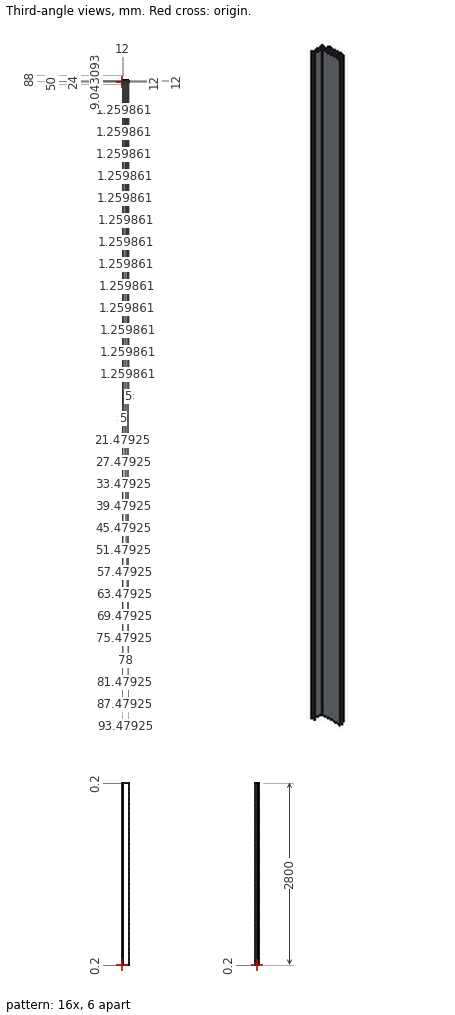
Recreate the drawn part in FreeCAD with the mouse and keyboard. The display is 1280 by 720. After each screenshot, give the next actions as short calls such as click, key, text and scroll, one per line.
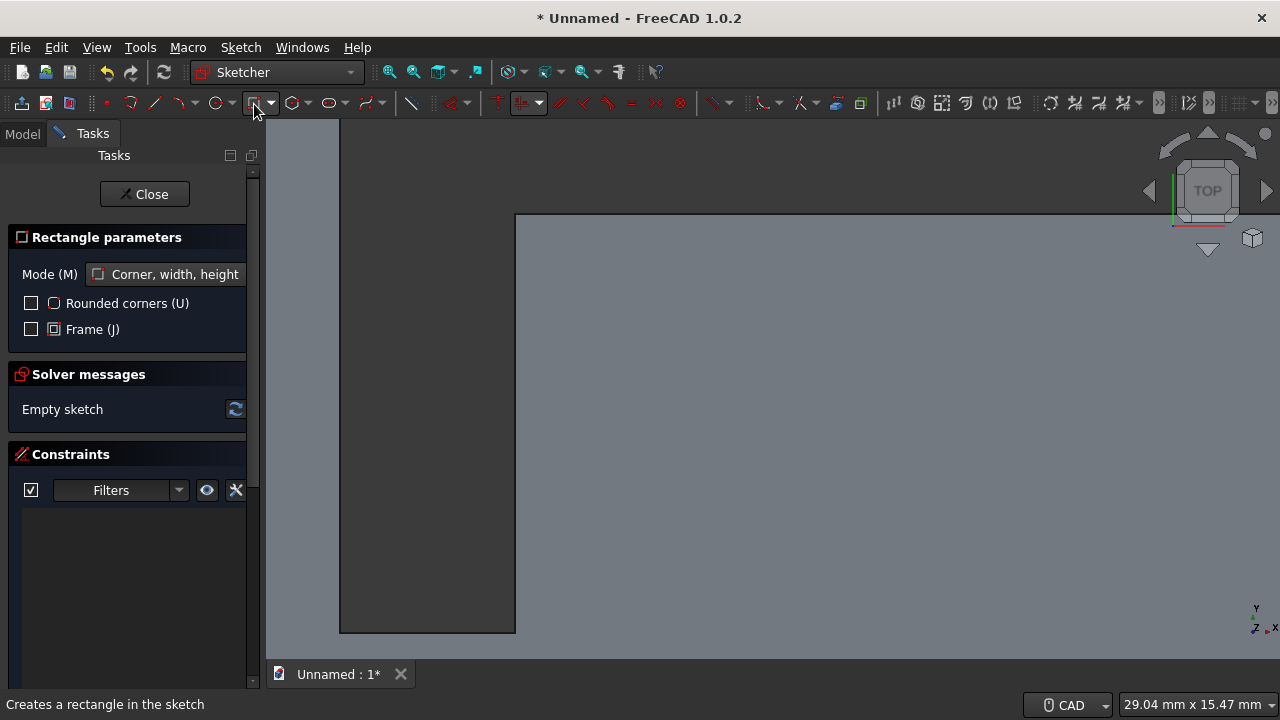
click(671, 214)
move(715, 530)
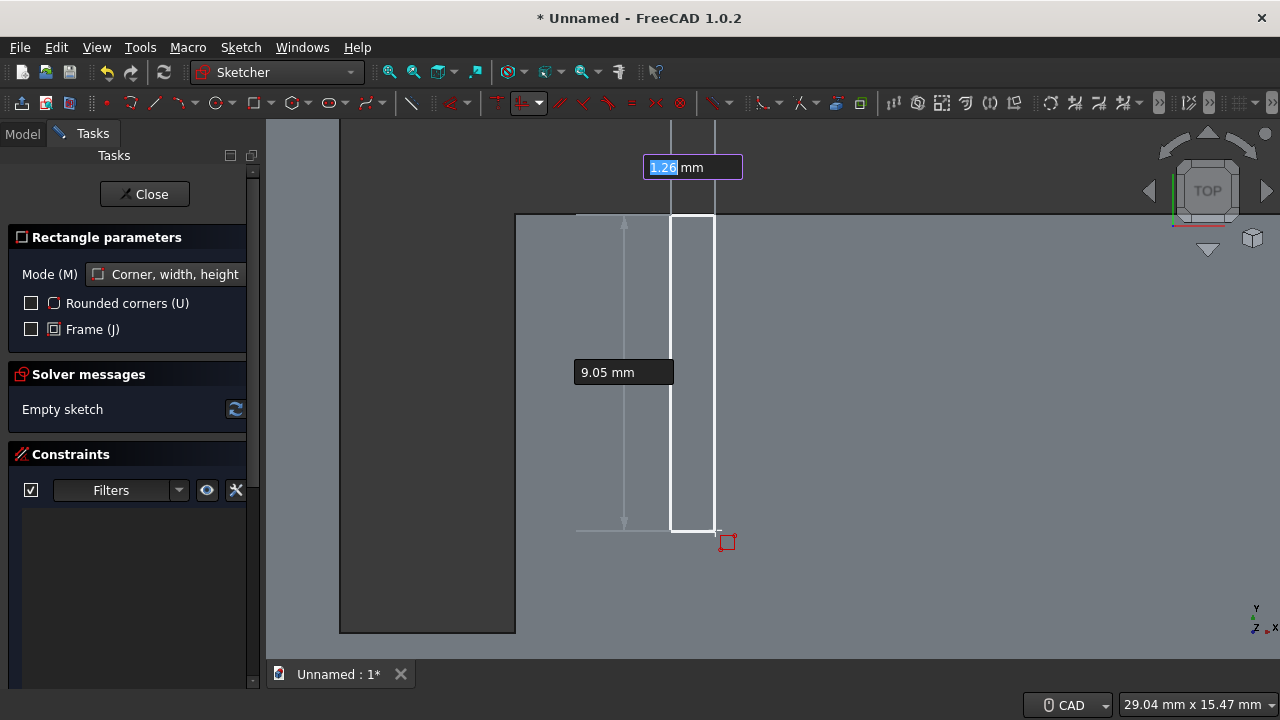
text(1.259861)
key(Tab)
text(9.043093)
key(Return)
key(Escape)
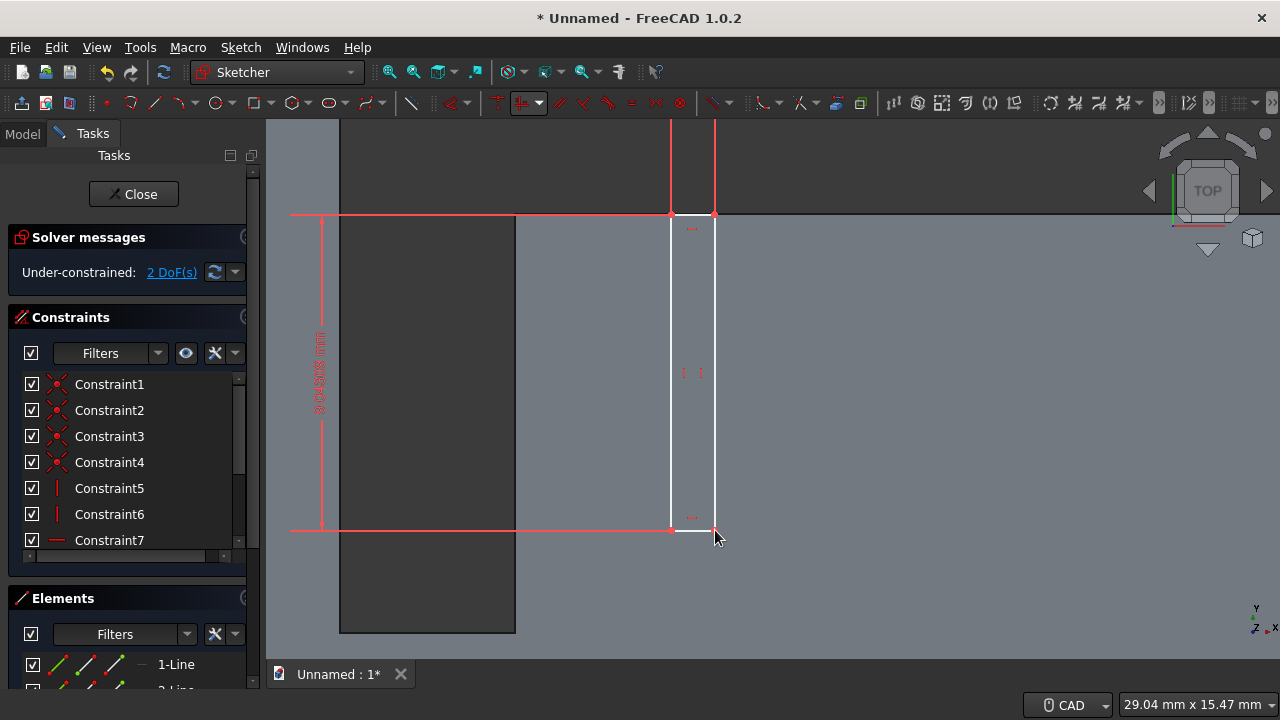
click(450, 104)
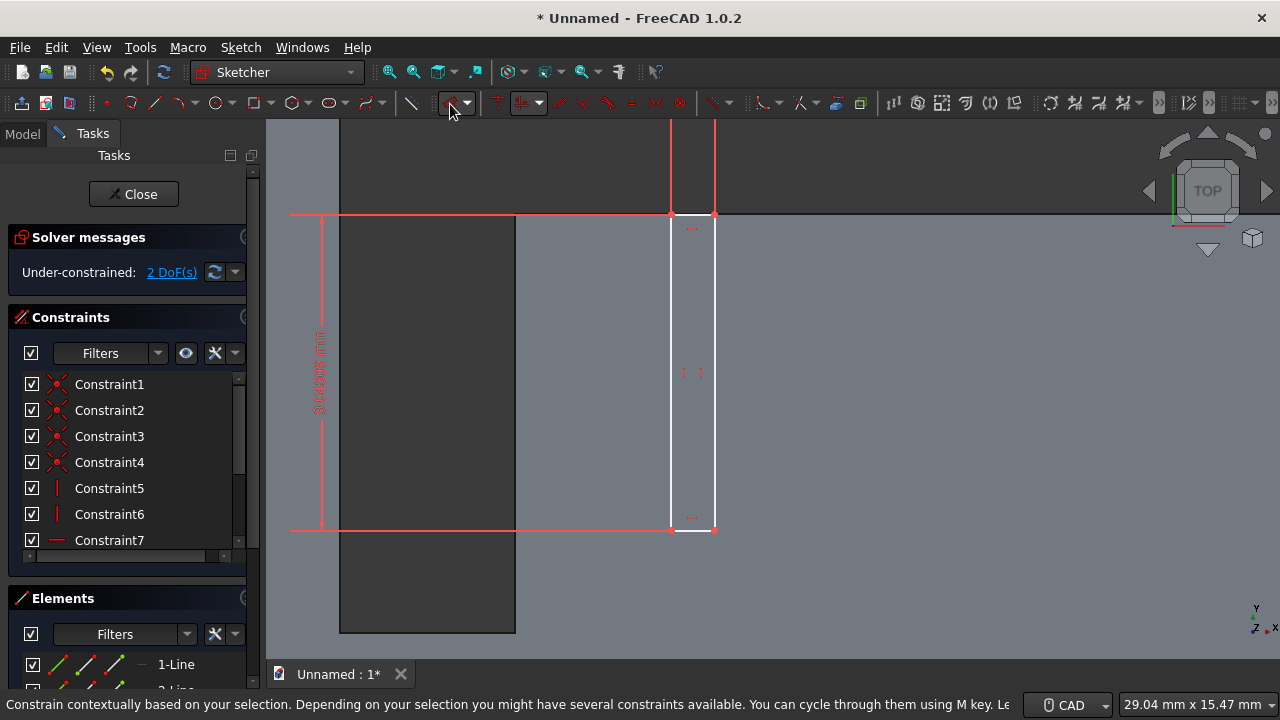
click(671, 215)
click(705, 569)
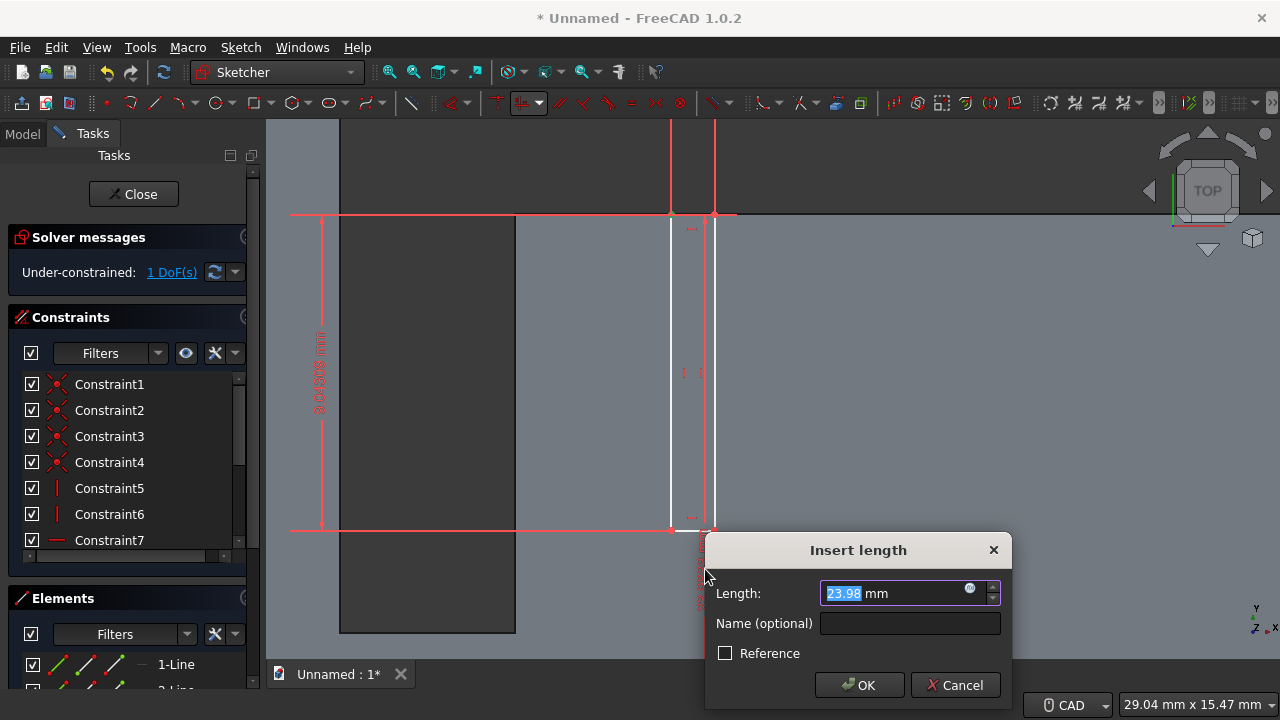
text(24)
key(Return)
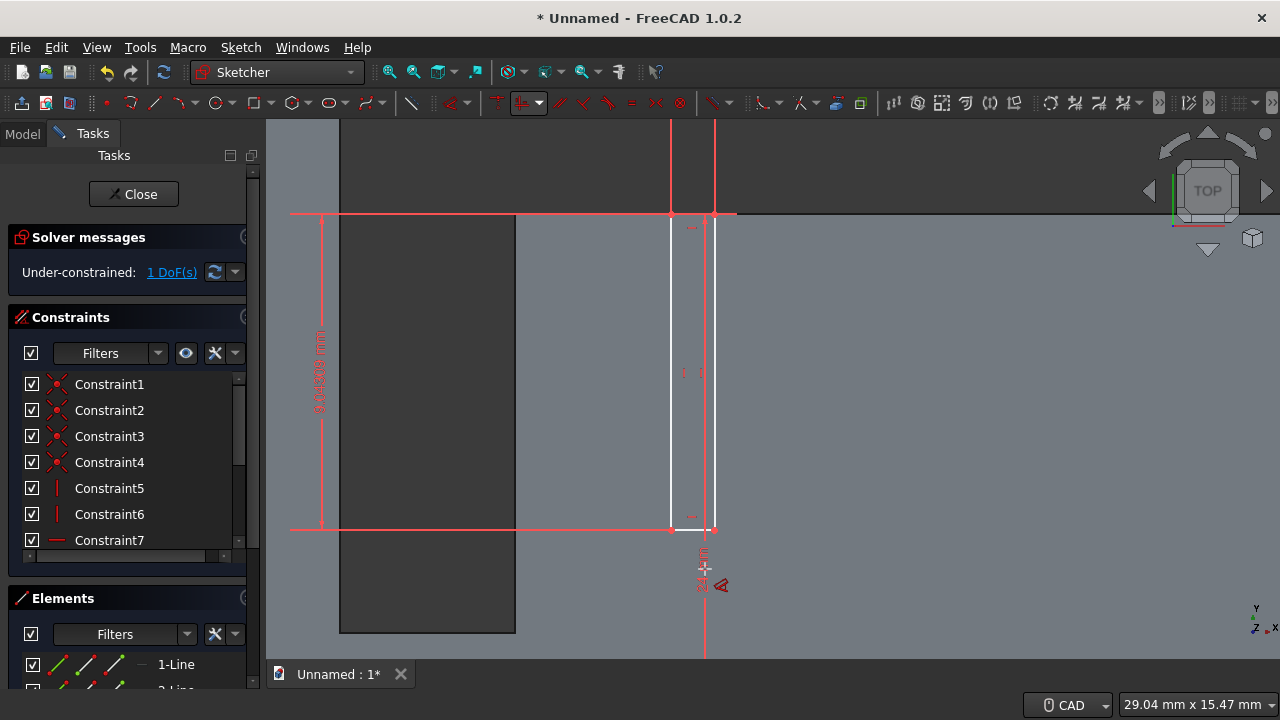
click(671, 214)
click(482, 180)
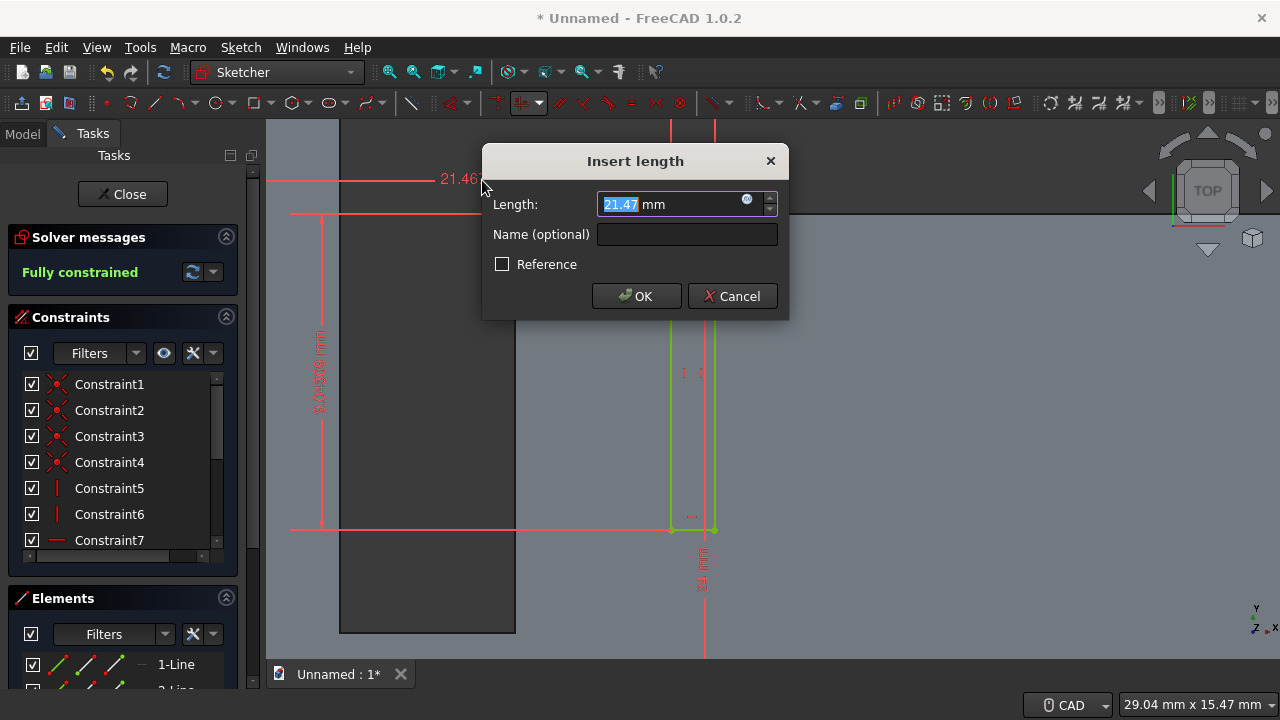
text(21.47925)
key(Return)
key(Escape)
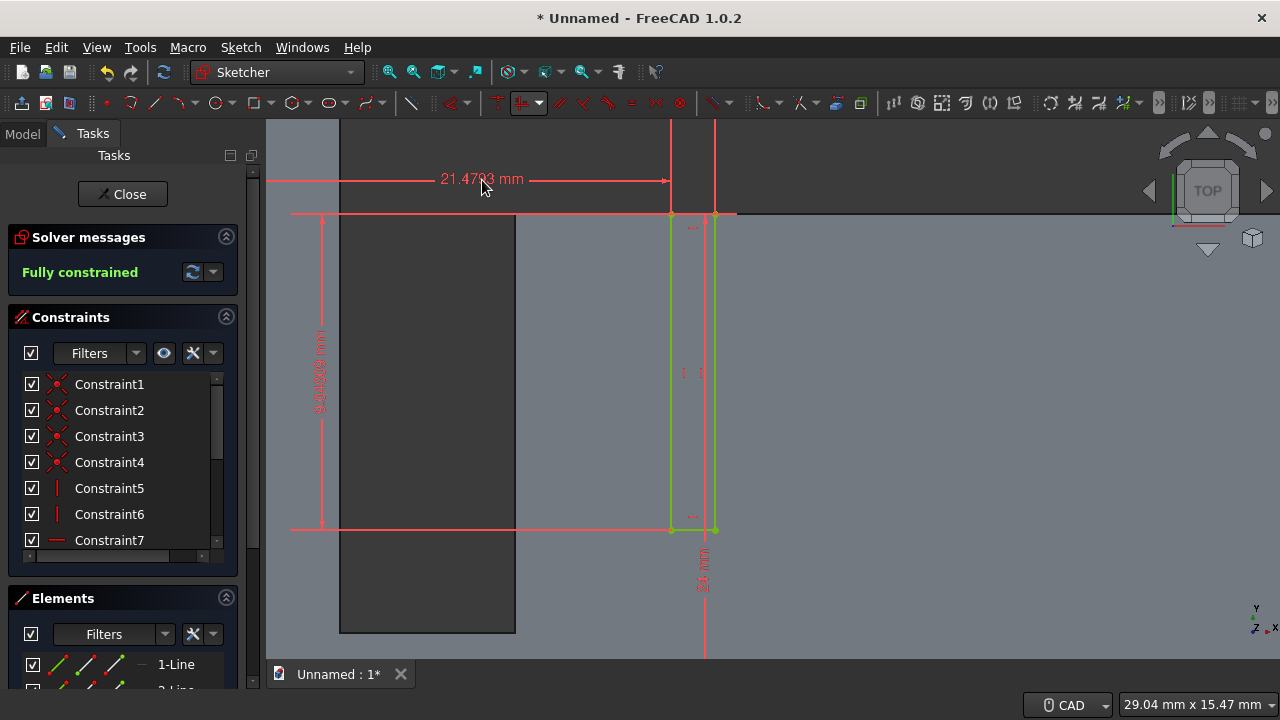
click(123, 194)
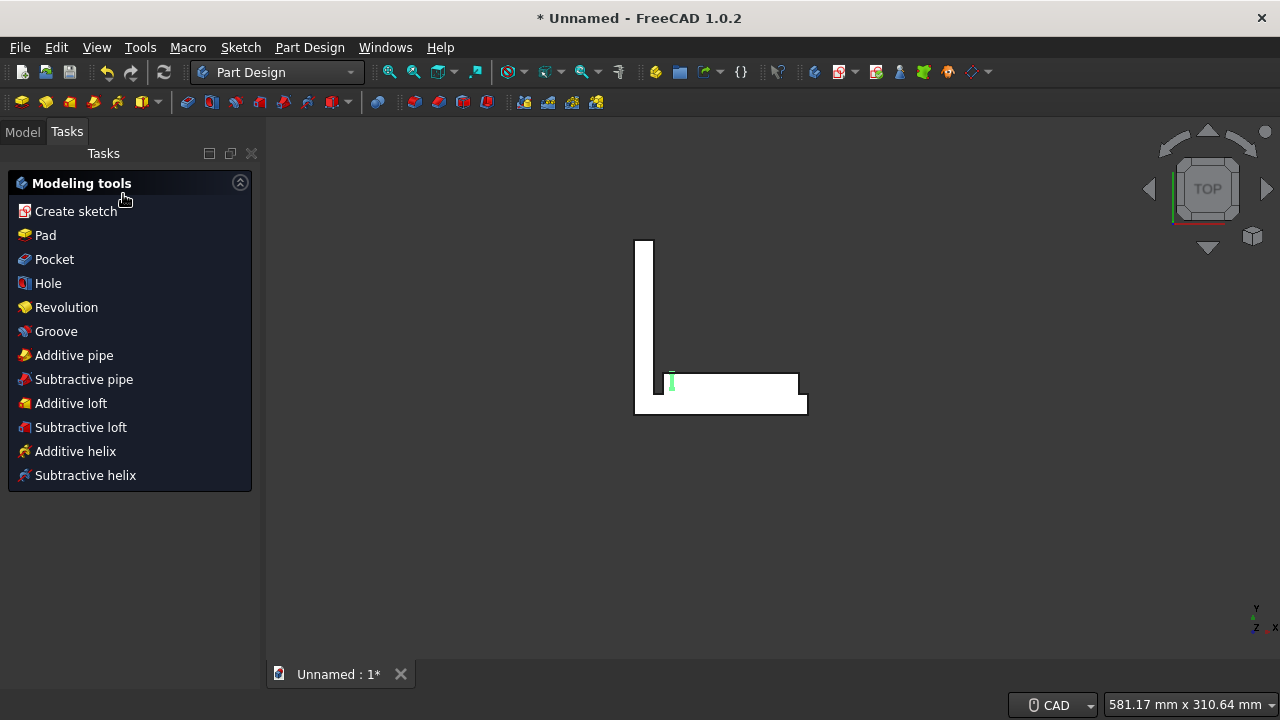
click(188, 102)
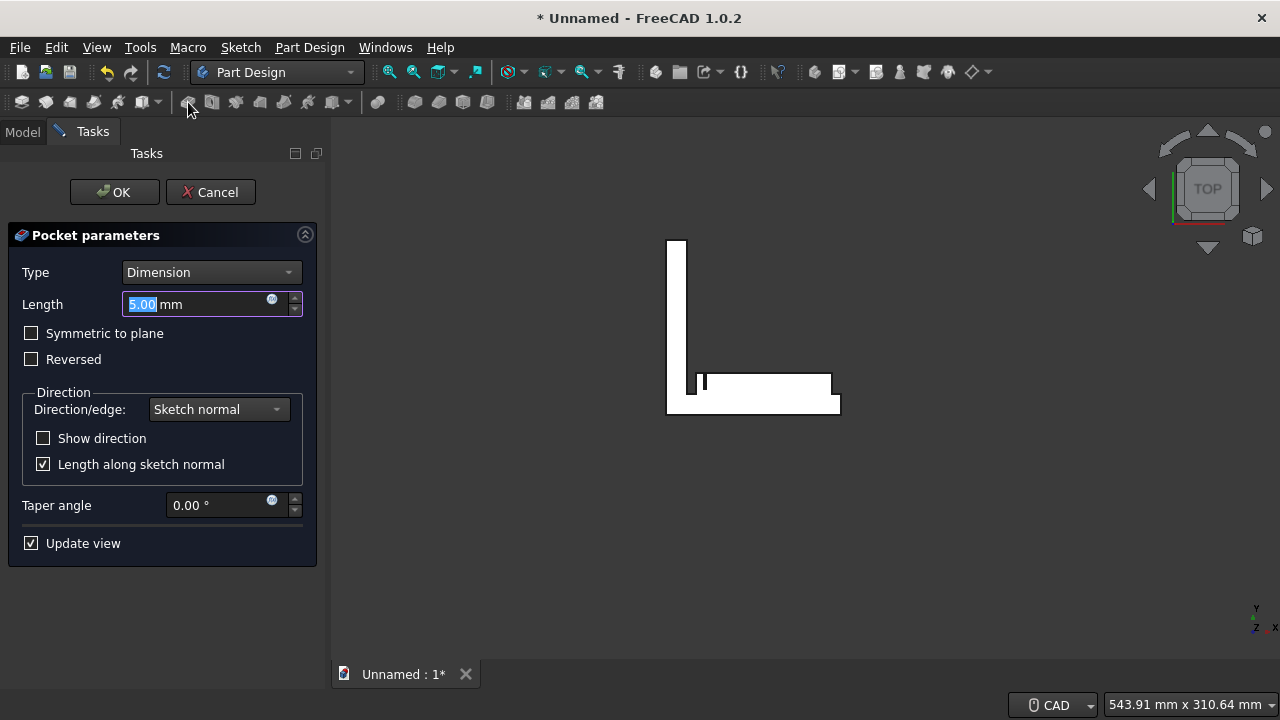
text(0.2)
key(Tab)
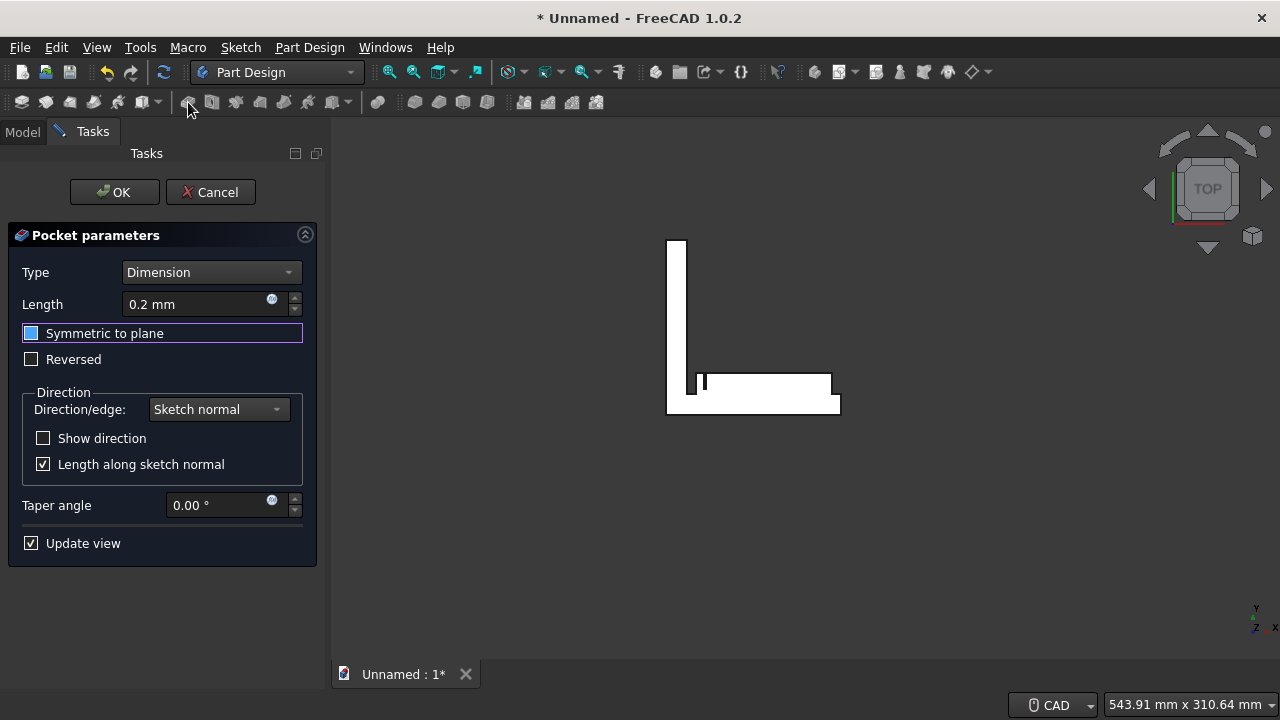
click(115, 192)